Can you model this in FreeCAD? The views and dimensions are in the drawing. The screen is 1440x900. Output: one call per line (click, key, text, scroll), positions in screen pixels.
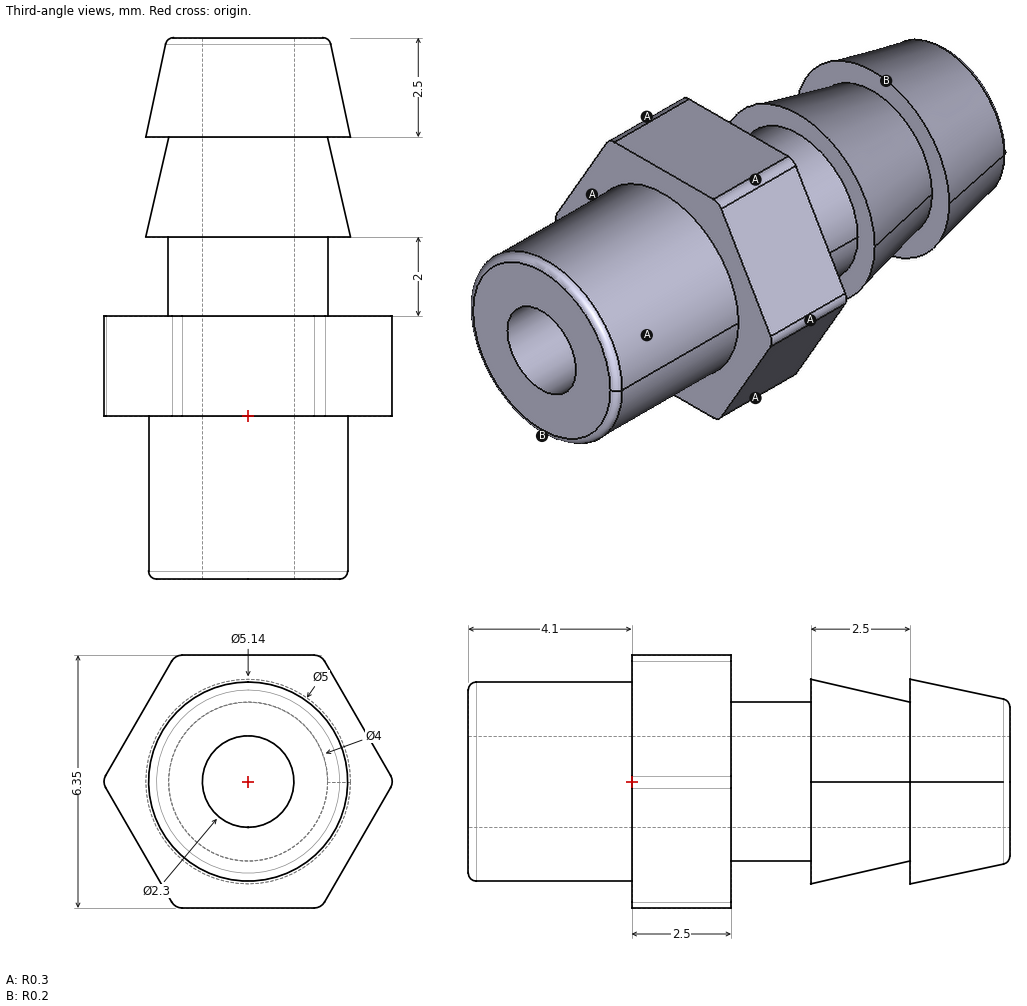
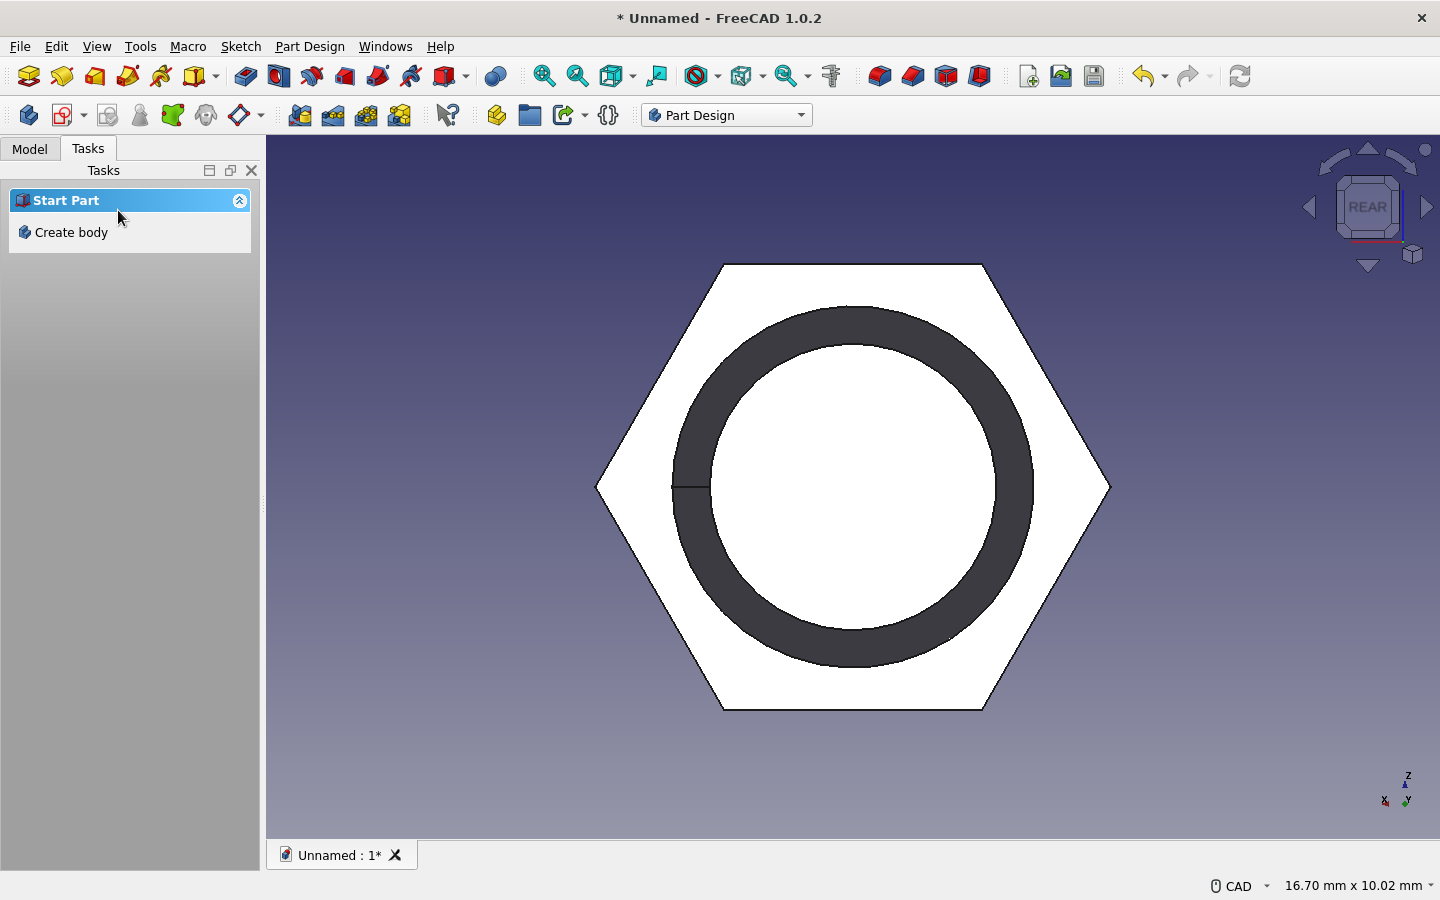
key(0)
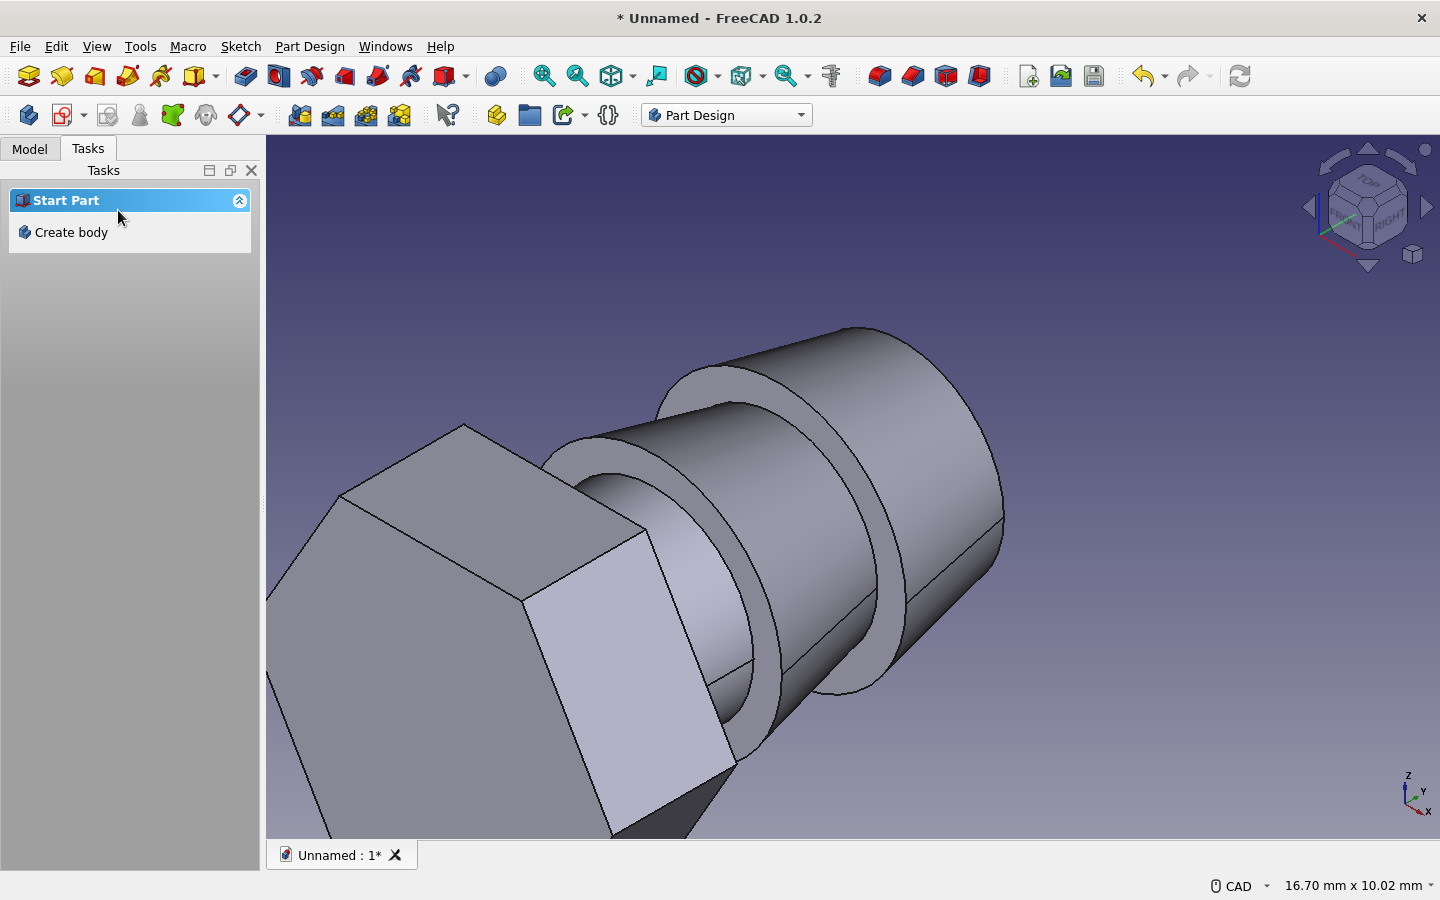
click(545, 76)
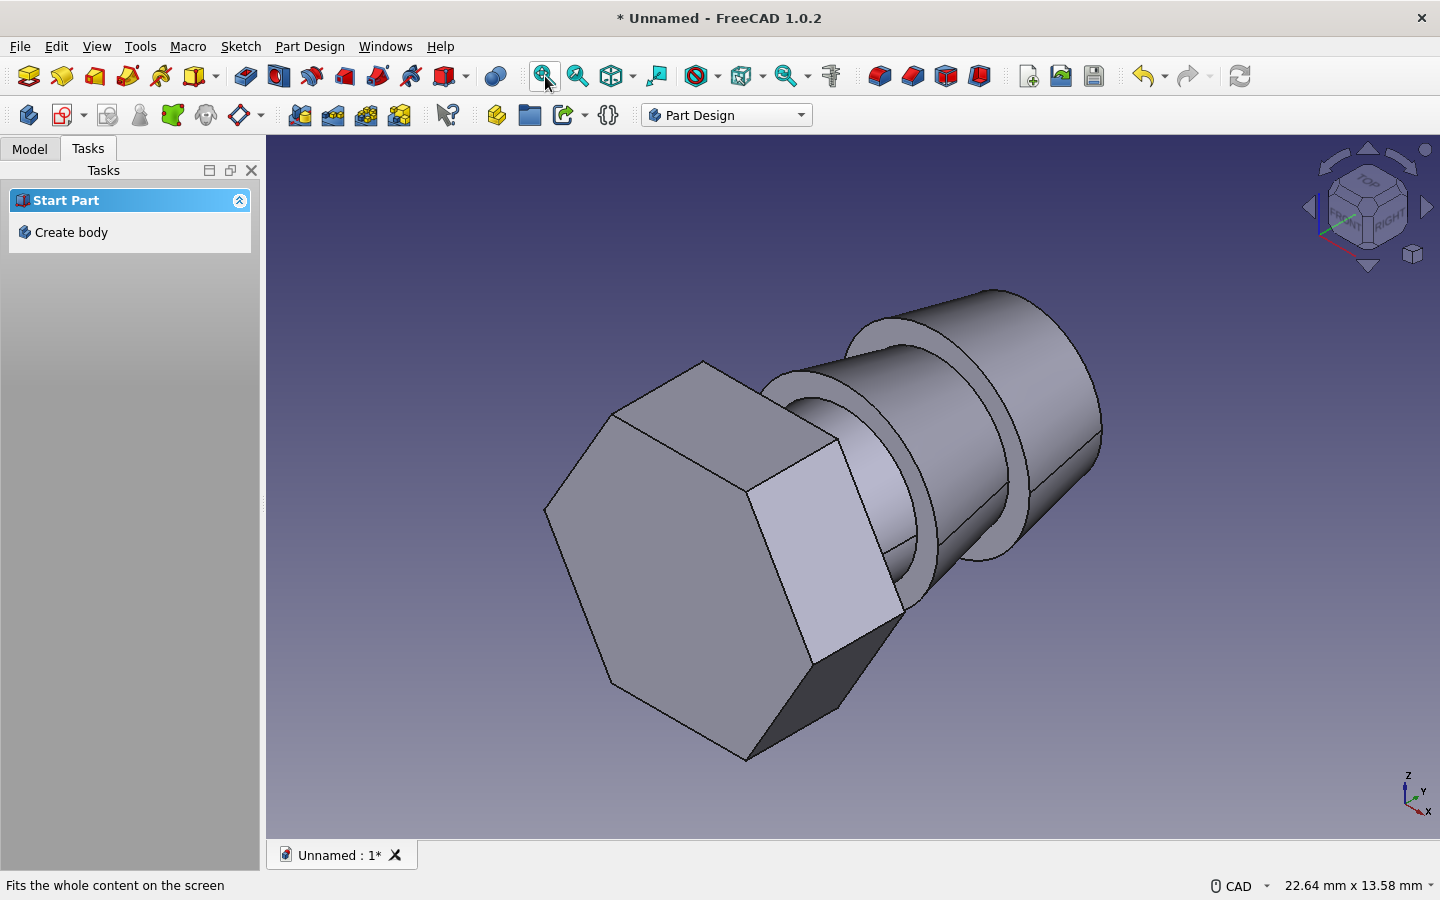
click(679, 587)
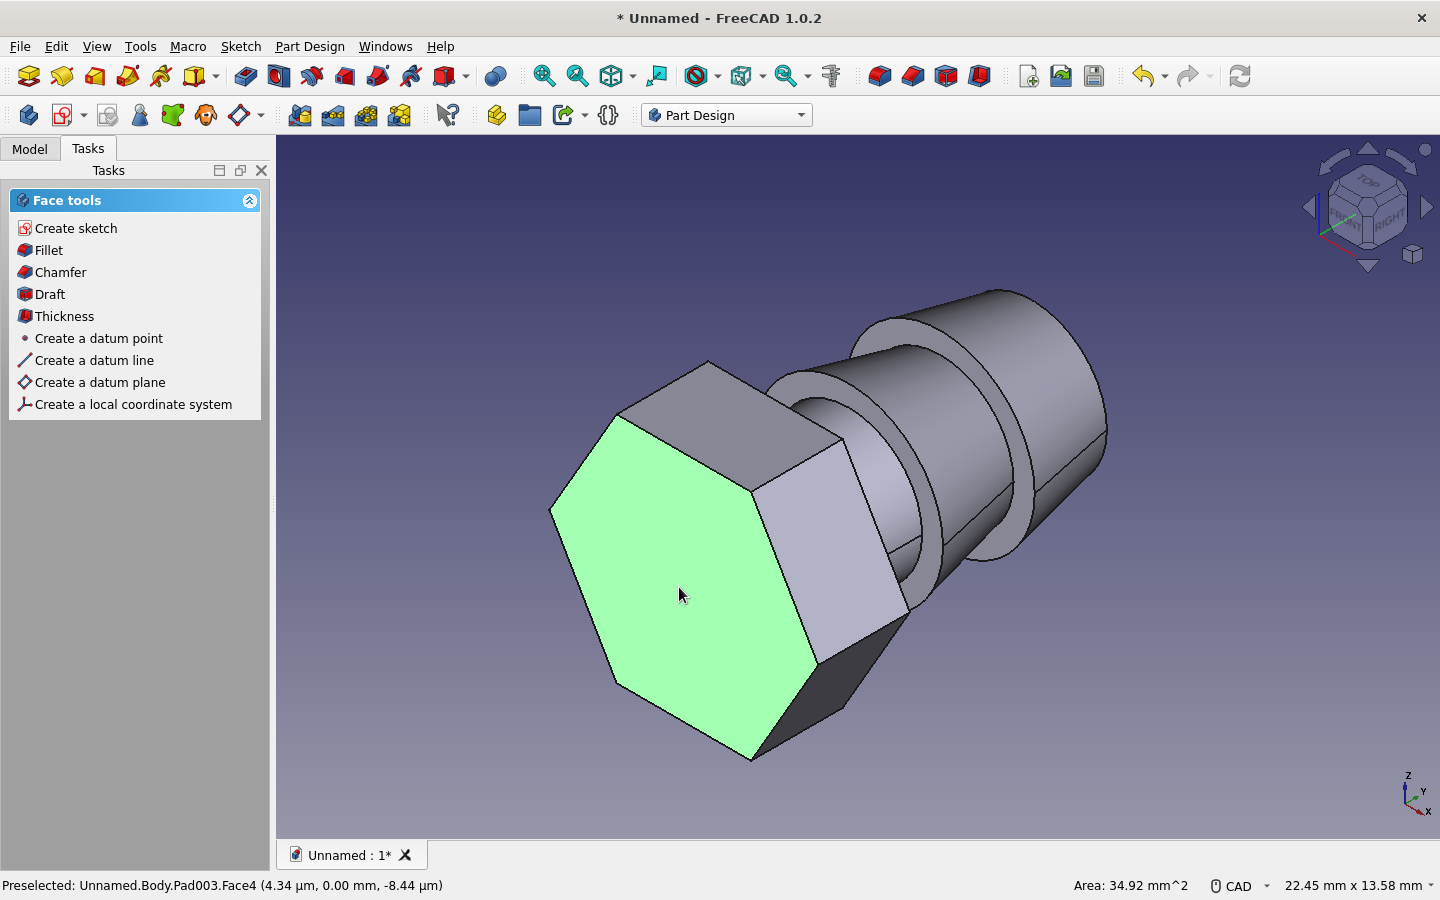
click(62, 116)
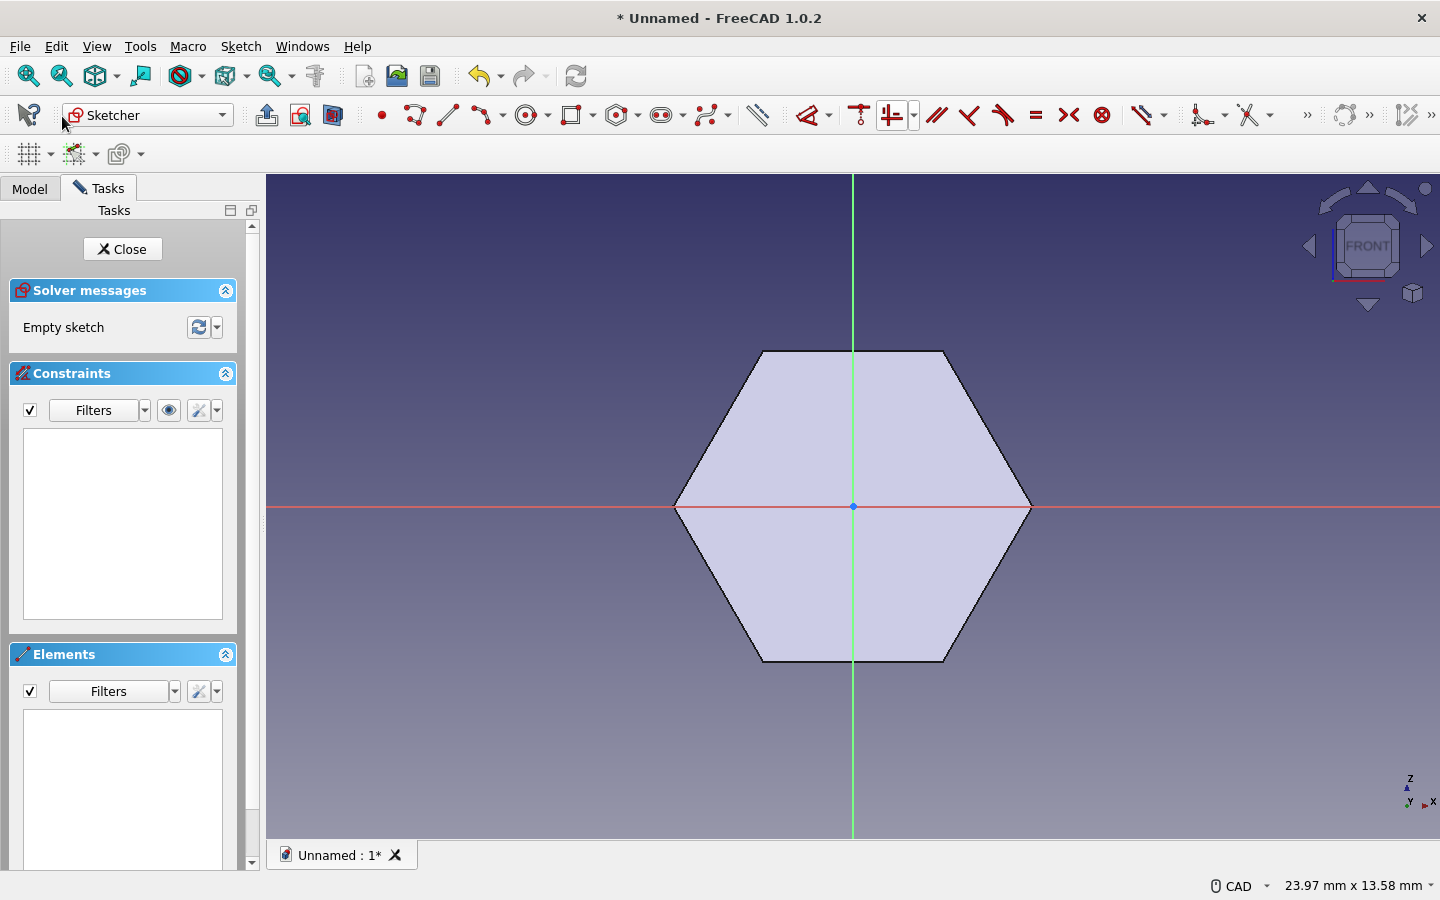
scroll(936, 507, up, 3)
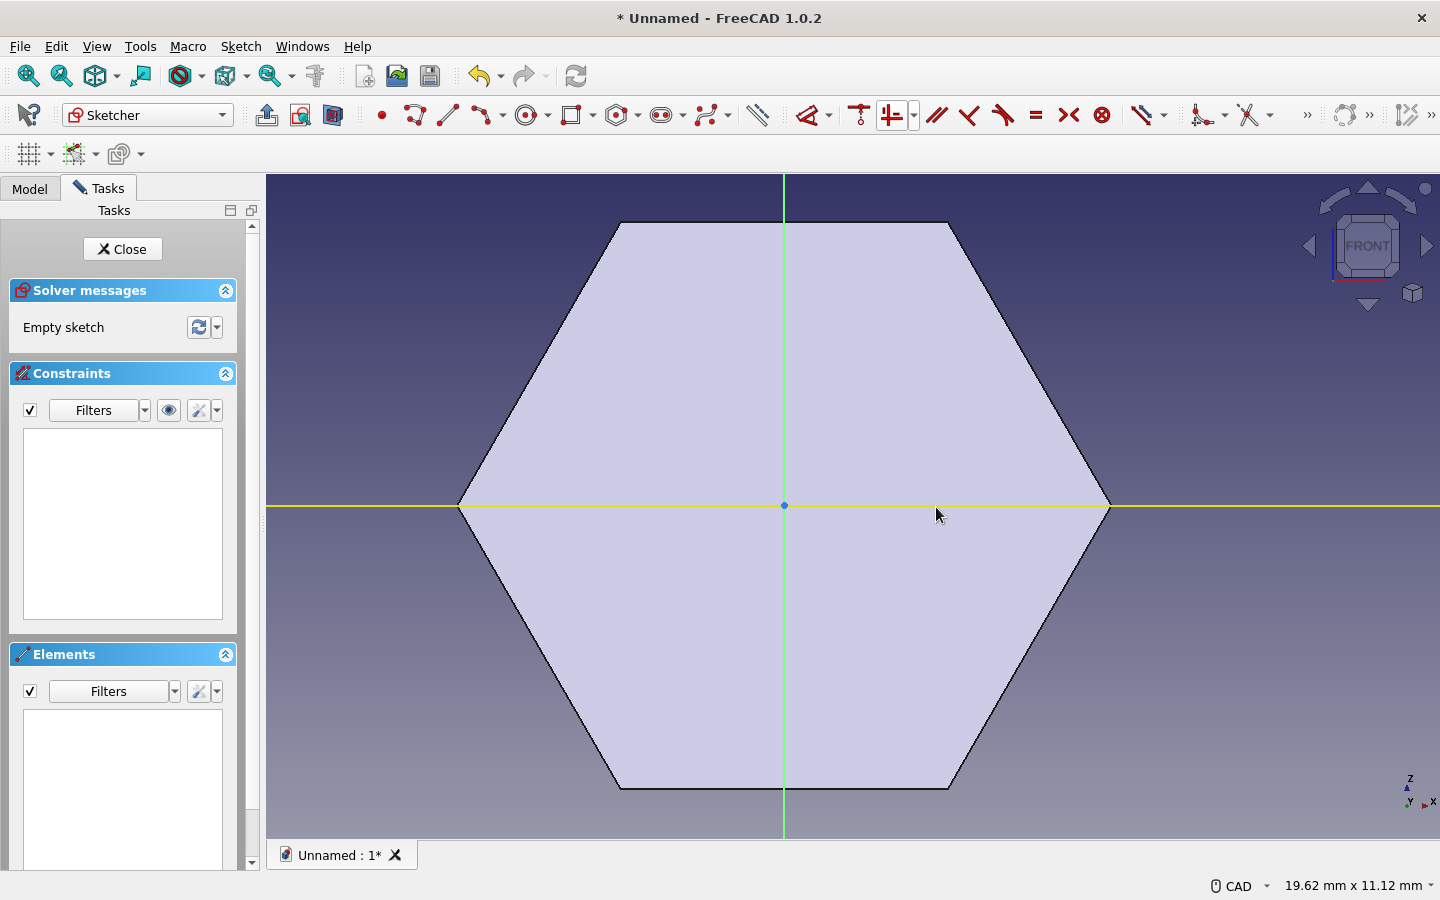
click(526, 116)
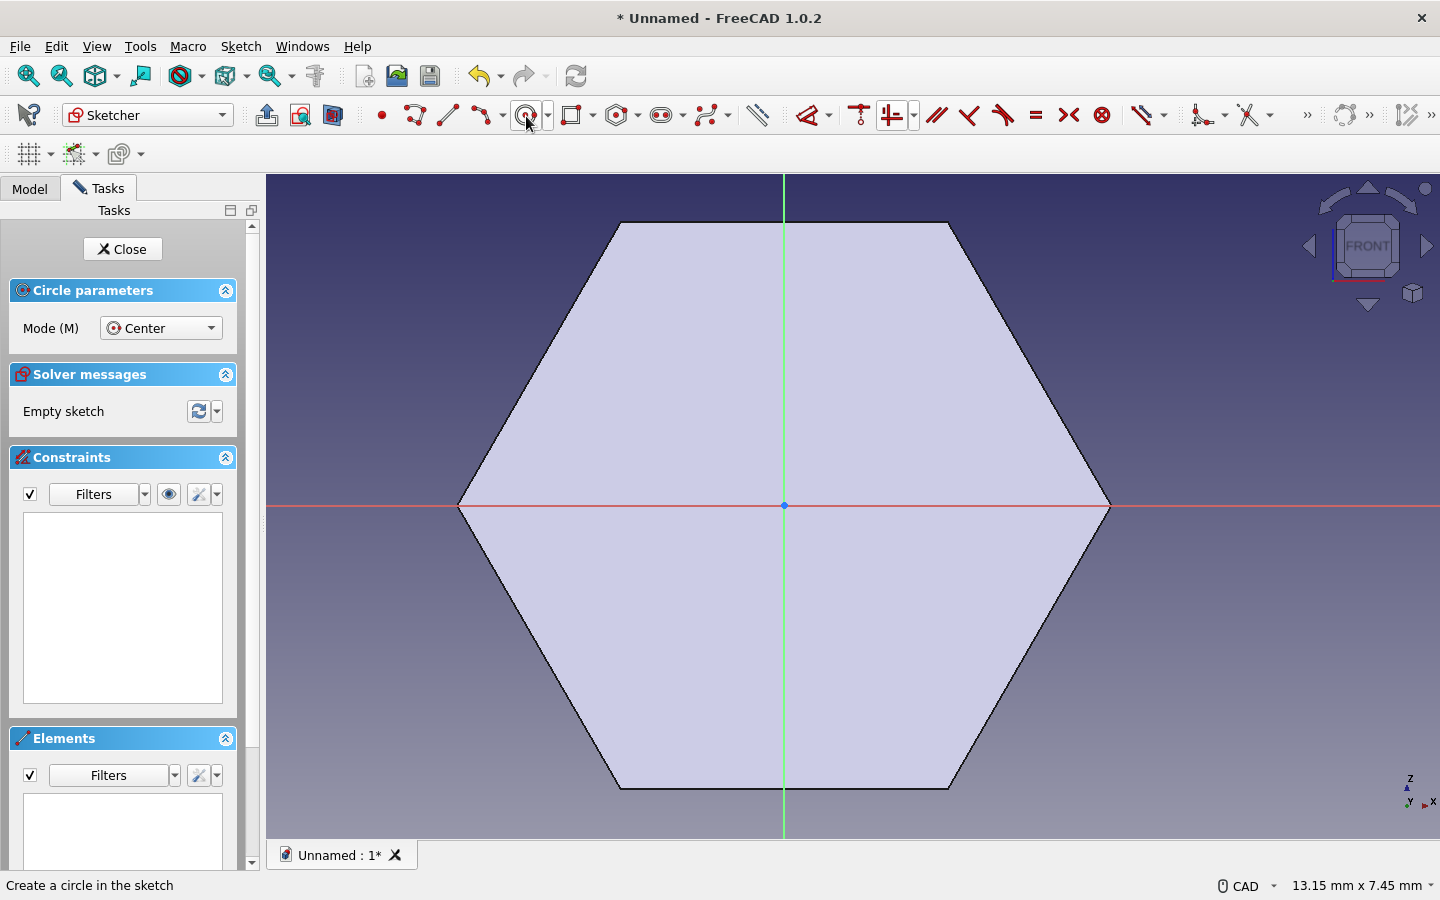
click(784, 506)
click(942, 348)